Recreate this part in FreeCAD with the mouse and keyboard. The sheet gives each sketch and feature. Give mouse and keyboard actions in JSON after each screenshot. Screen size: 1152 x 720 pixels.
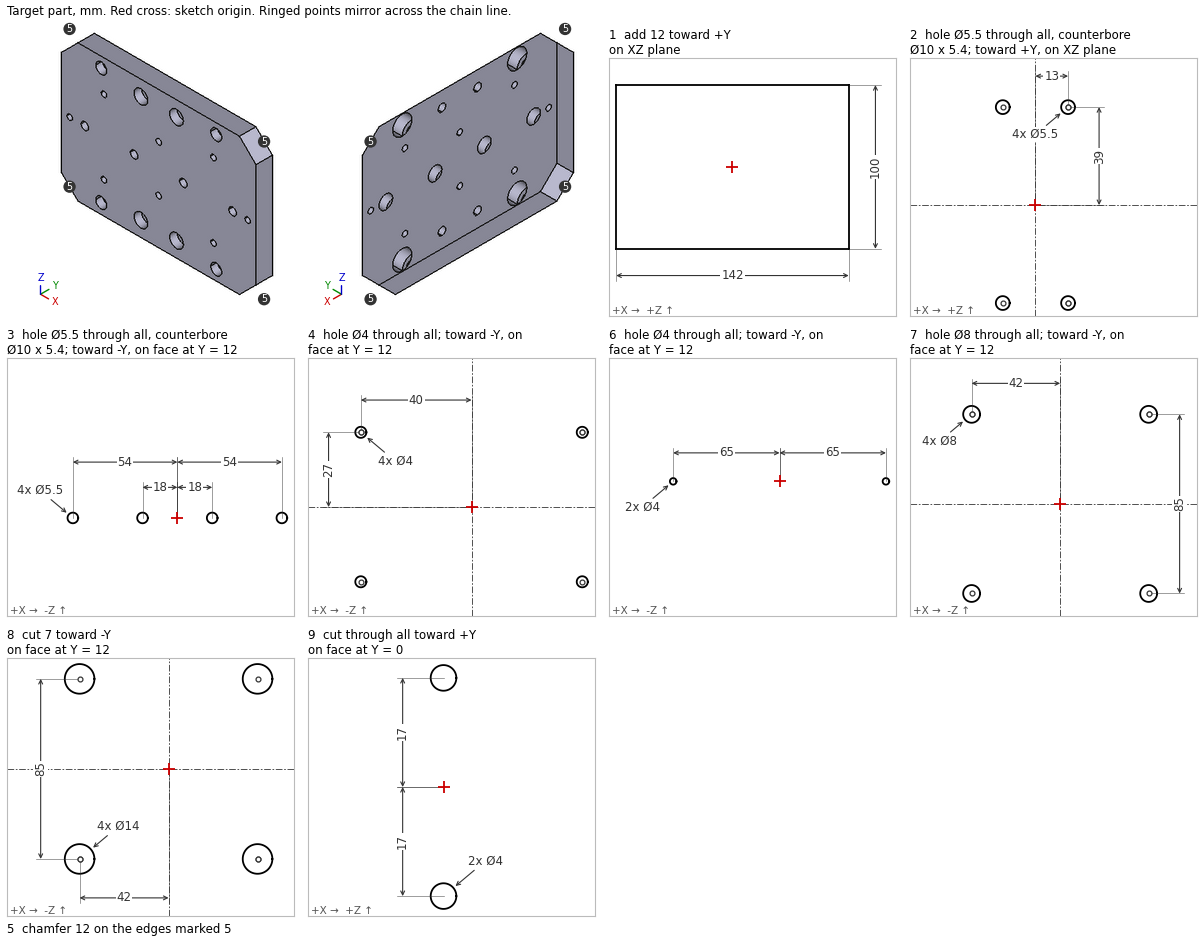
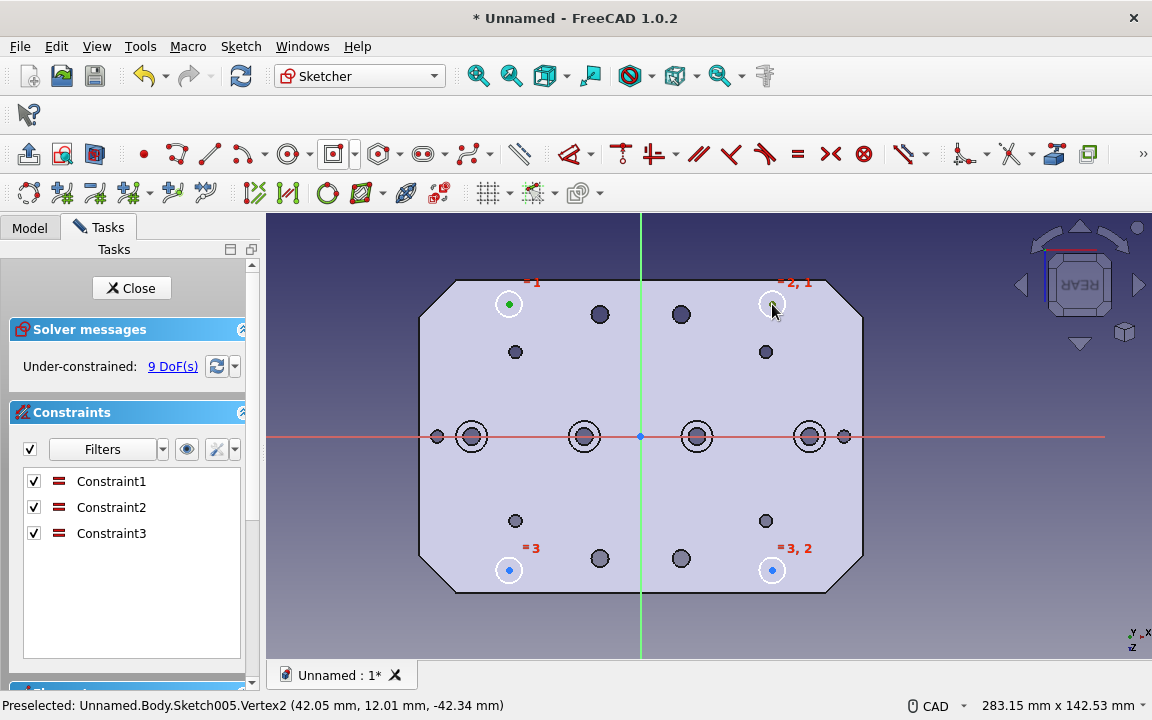
{"action": "left_click", "coordinate": [641, 603]}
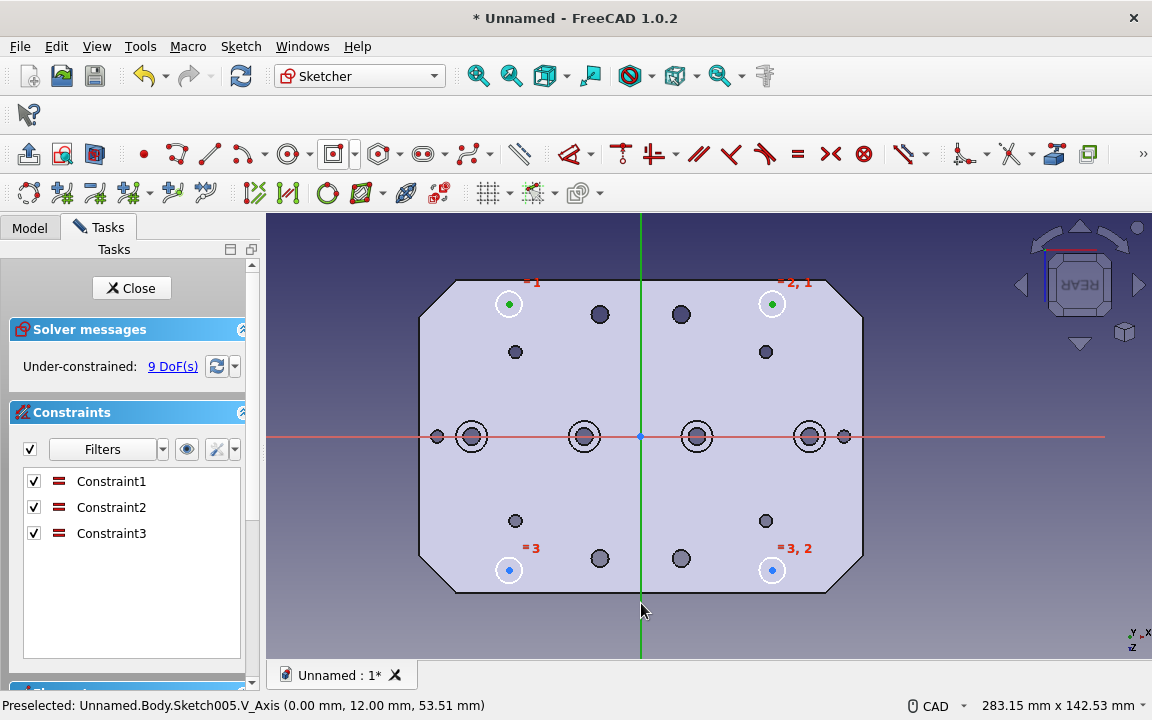
{"action": "left_click", "coordinate": [831, 154]}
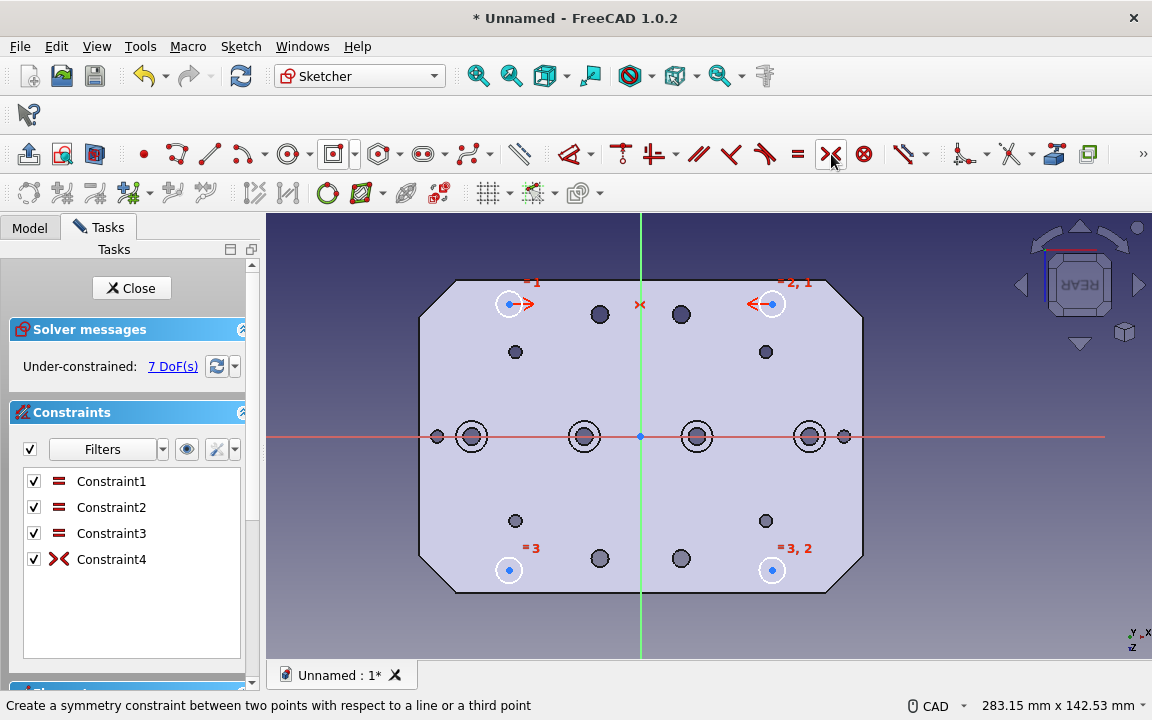
{"action": "left_click", "coordinate": [772, 304]}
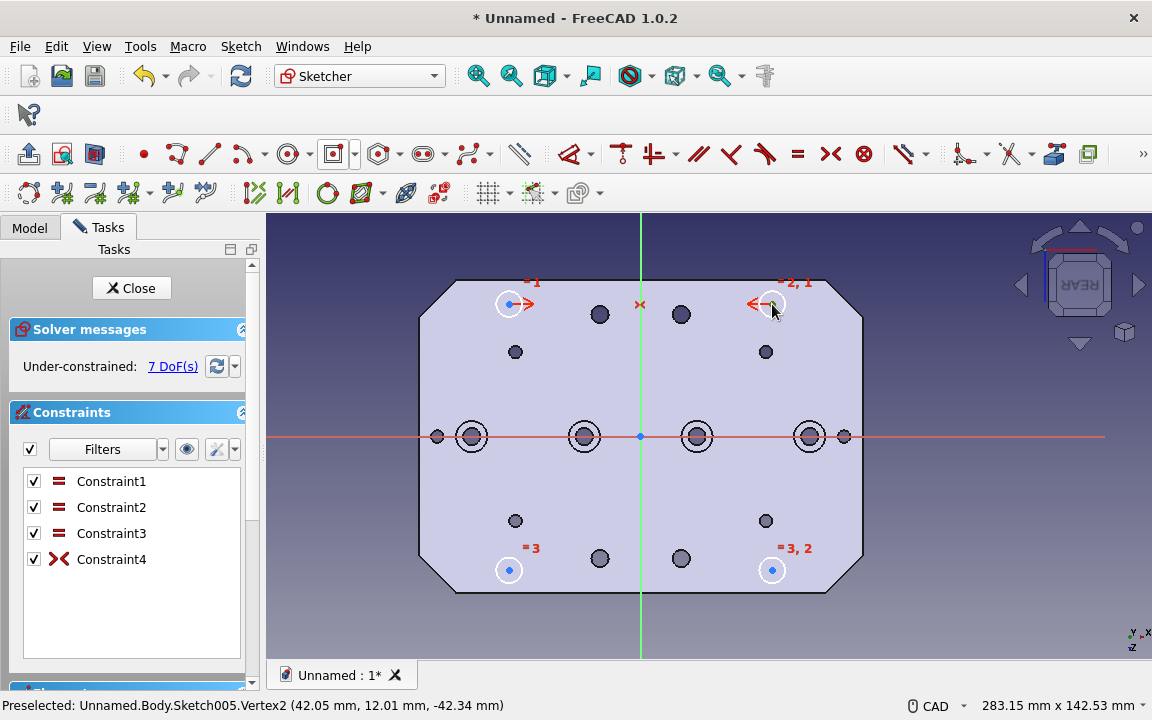
{"action": "left_click", "coordinate": [772, 570]}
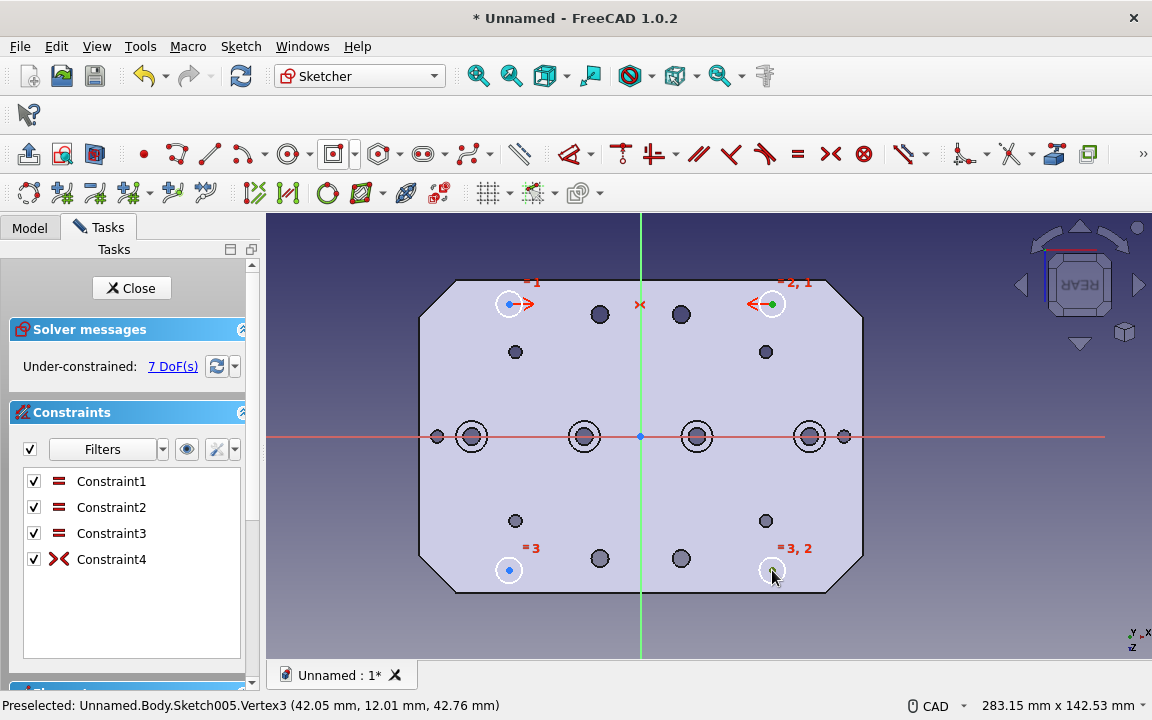
{"action": "left_click", "coordinate": [344, 437]}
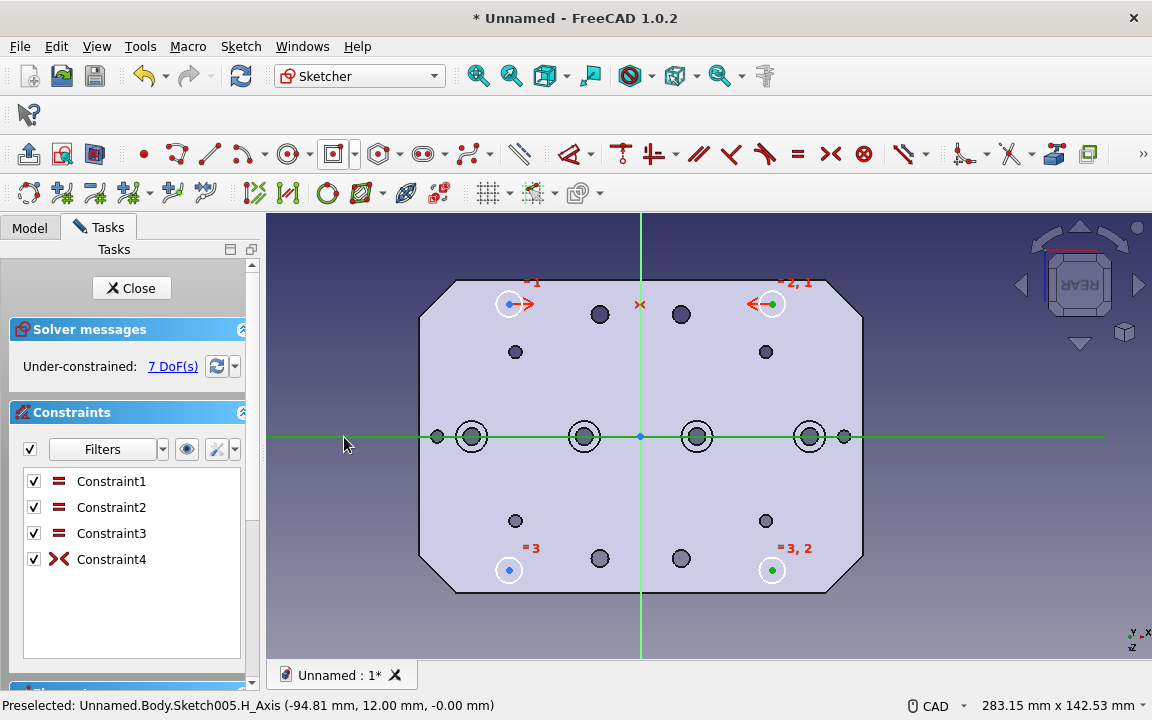
{"action": "left_click", "coordinate": [831, 154]}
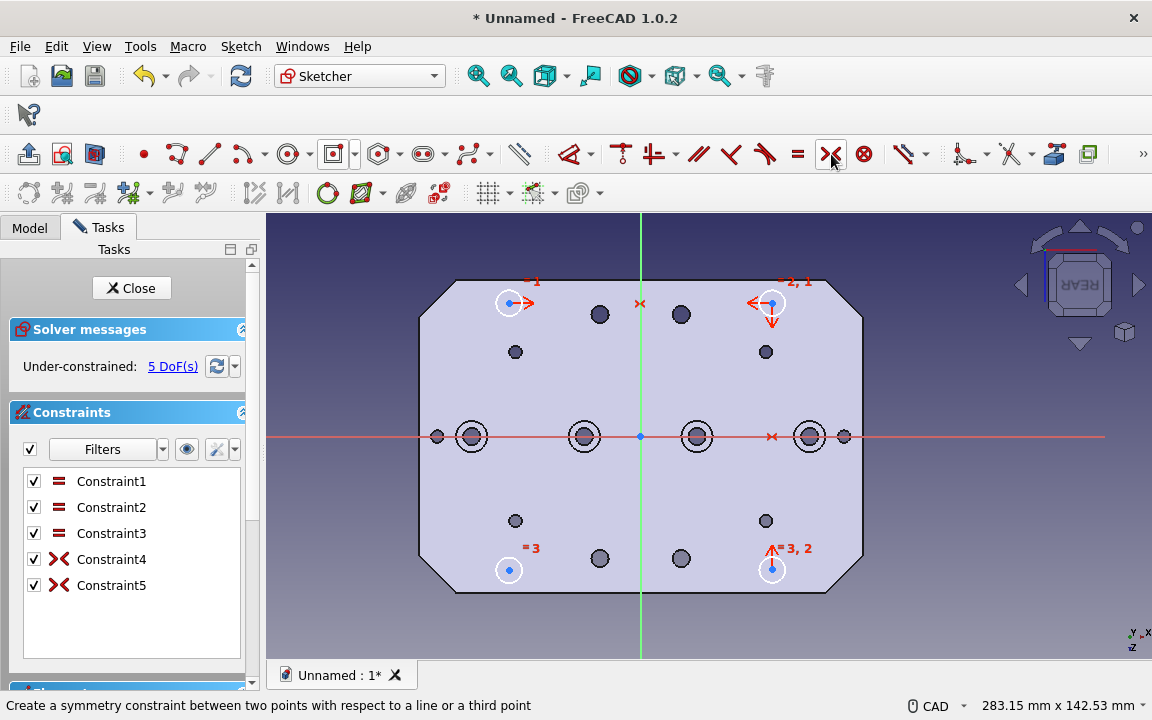
{"action": "left_click", "coordinate": [509, 303]}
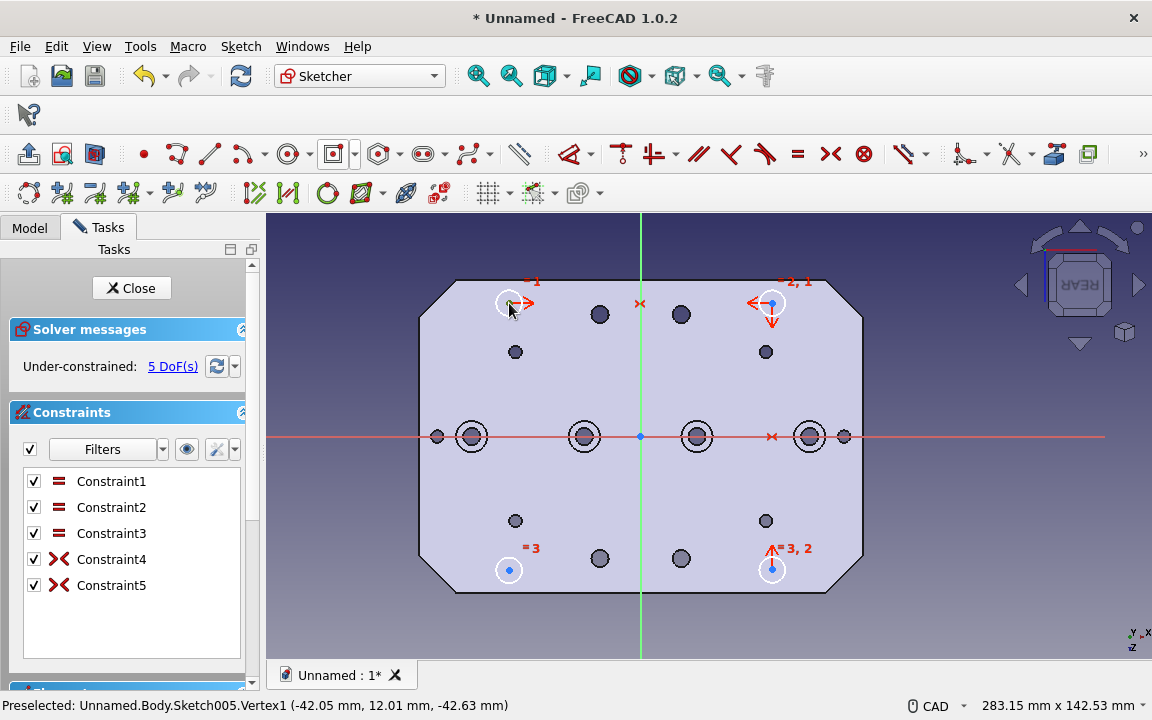
{"action": "left_click", "coordinate": [509, 570]}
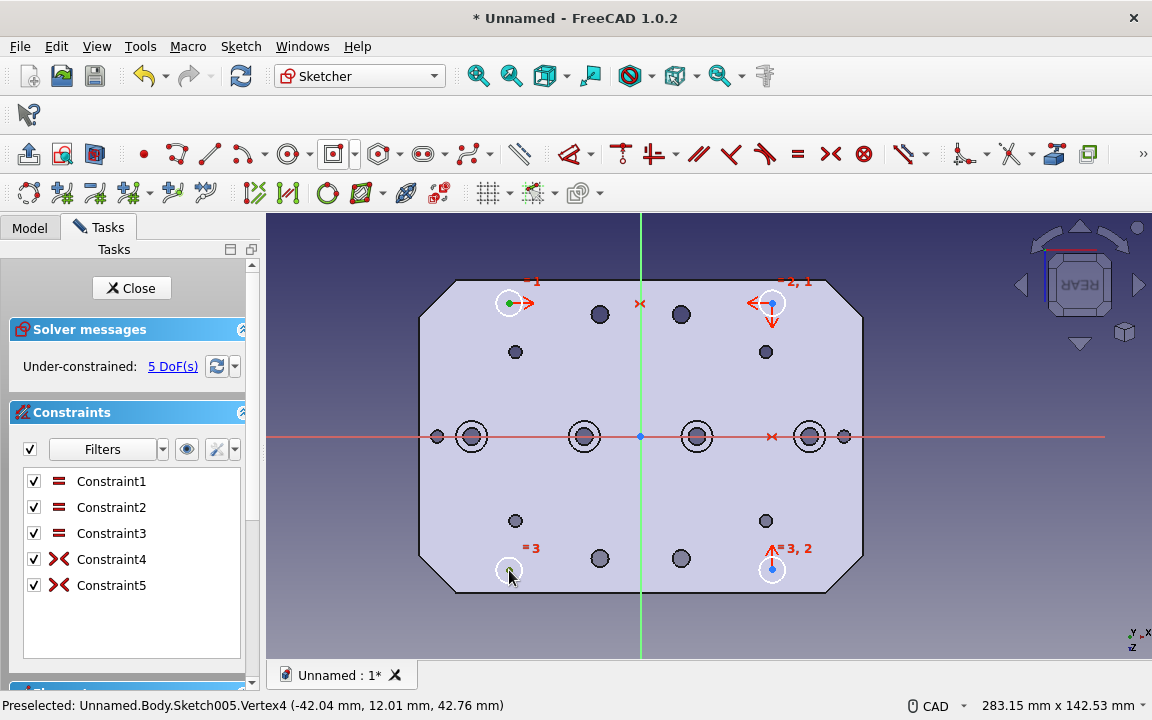
{"action": "left_click", "coordinate": [344, 437]}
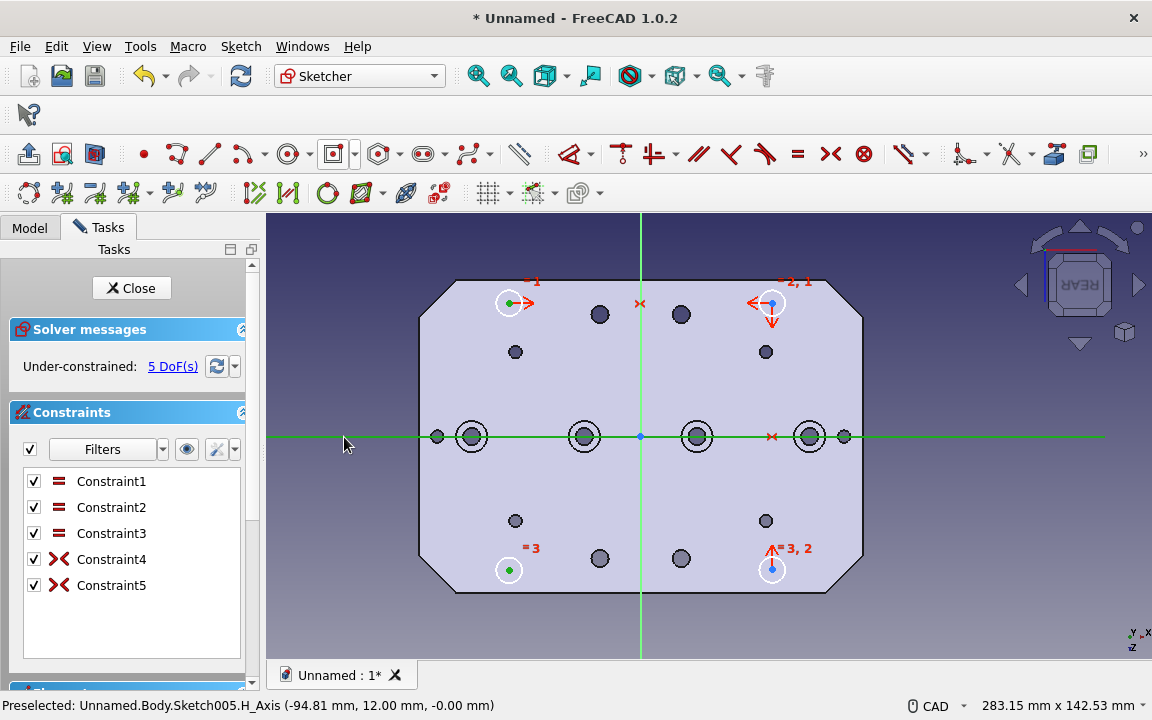
{"action": "left_click", "coordinate": [831, 154]}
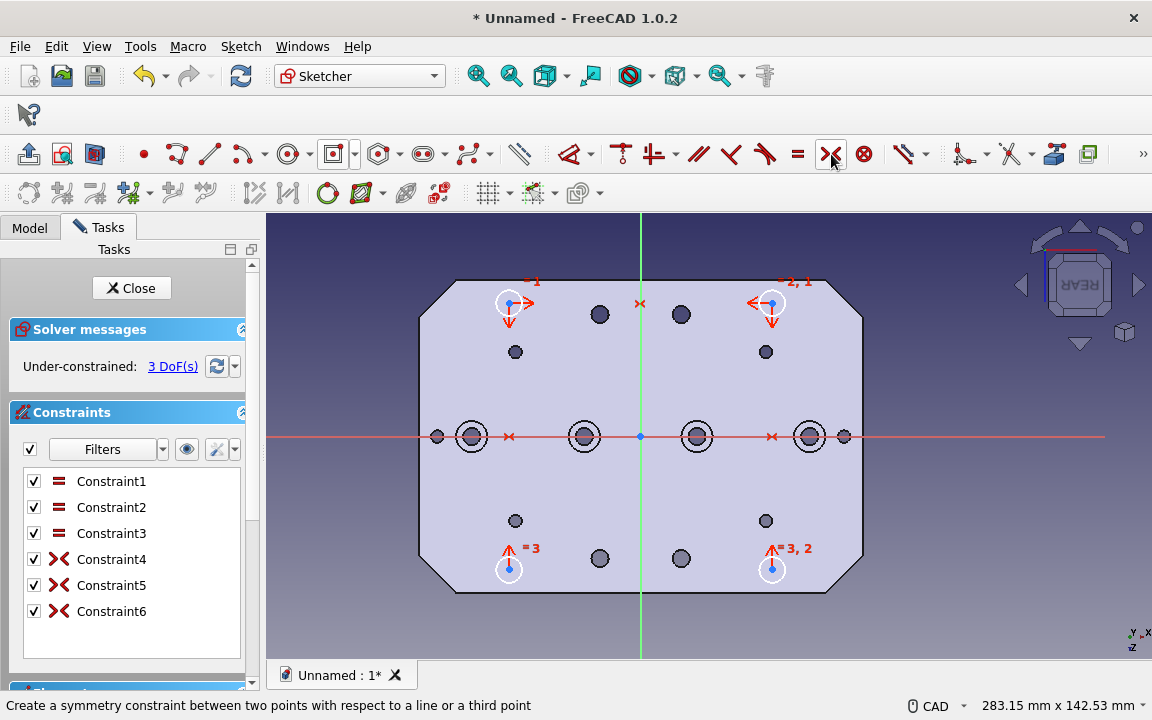
{"action": "left_click", "coordinate": [568, 154]}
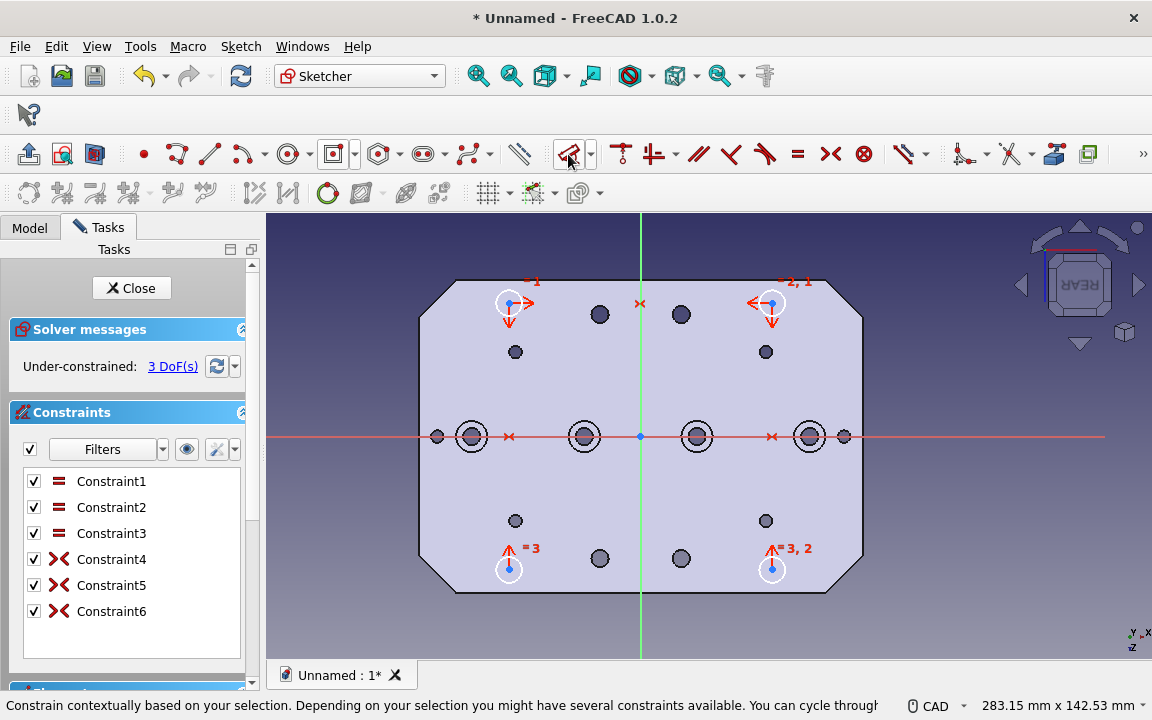
{"action": "scroll", "coordinate": [518, 294], "scroll_direction": "up", "scroll_amount": 3}